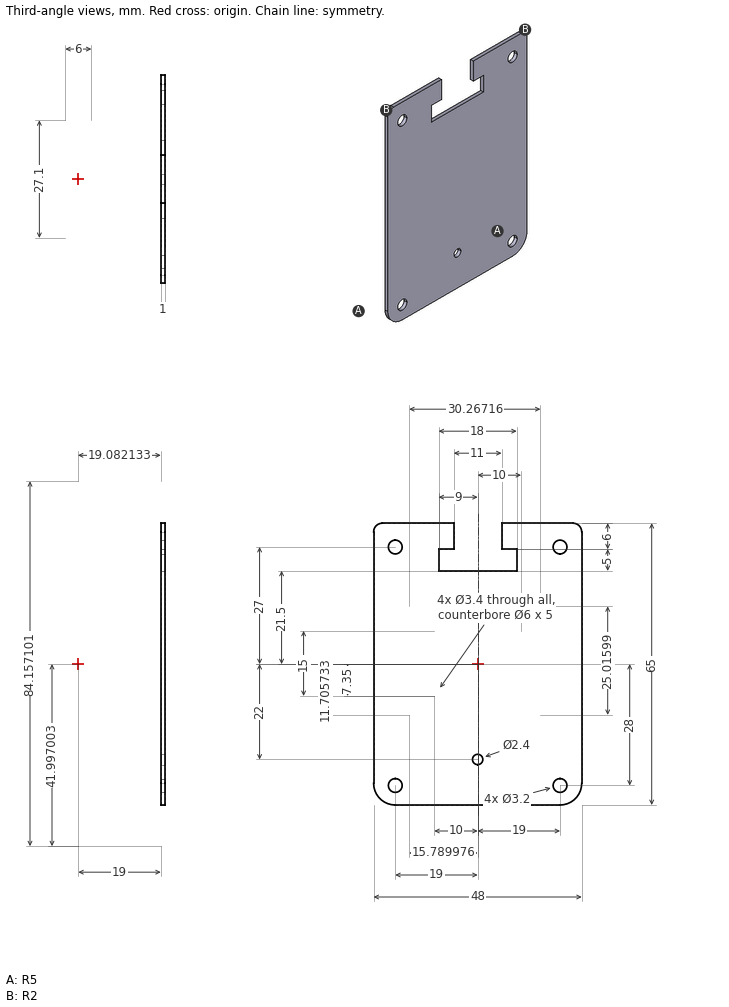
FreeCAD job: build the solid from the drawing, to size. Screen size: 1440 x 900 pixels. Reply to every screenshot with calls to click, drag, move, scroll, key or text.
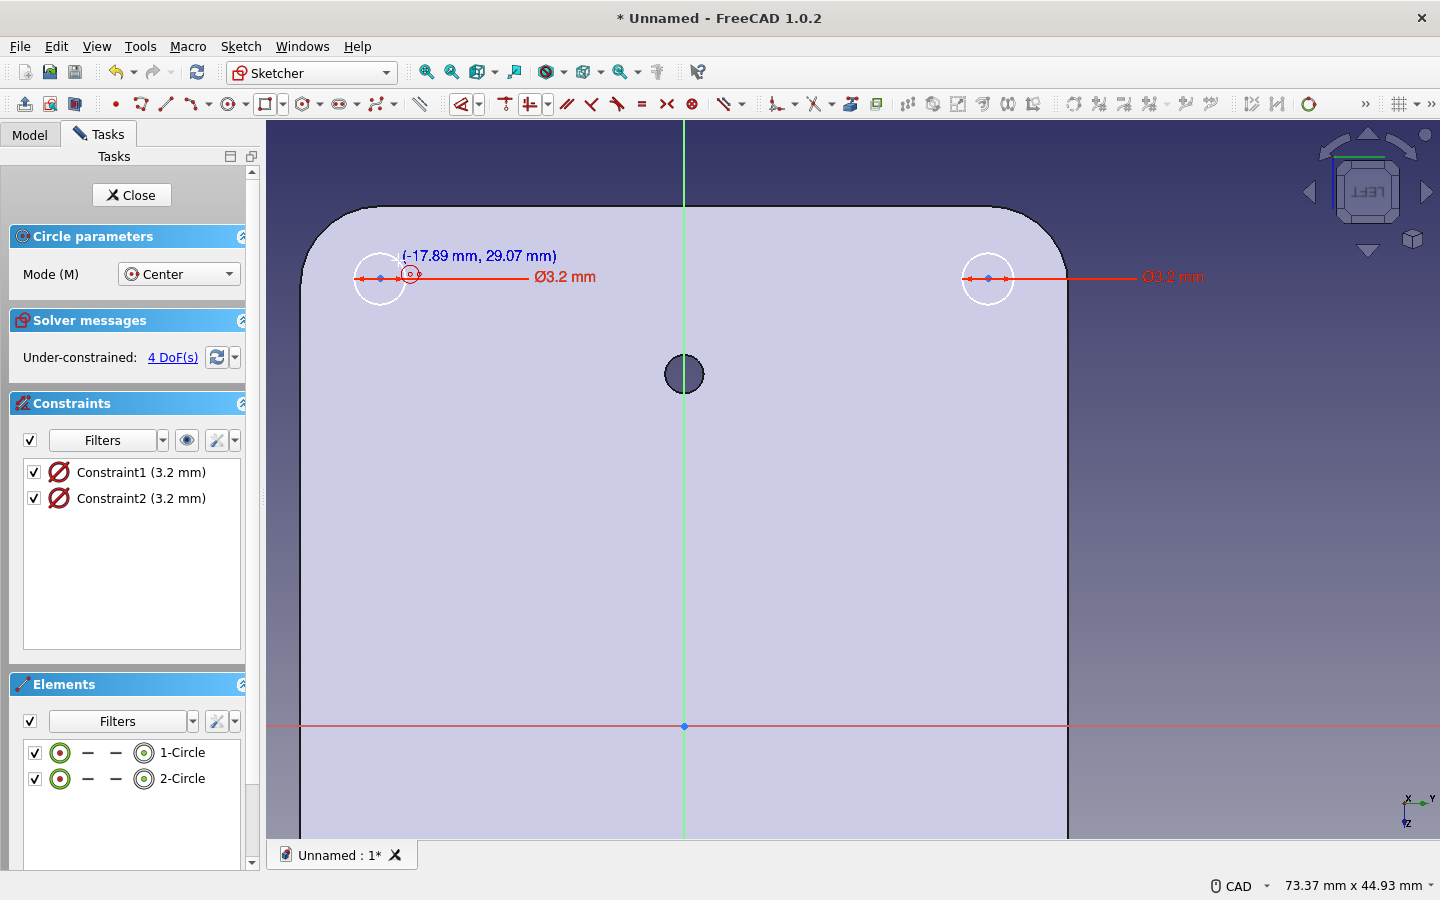
scroll(906, 189, down, 3)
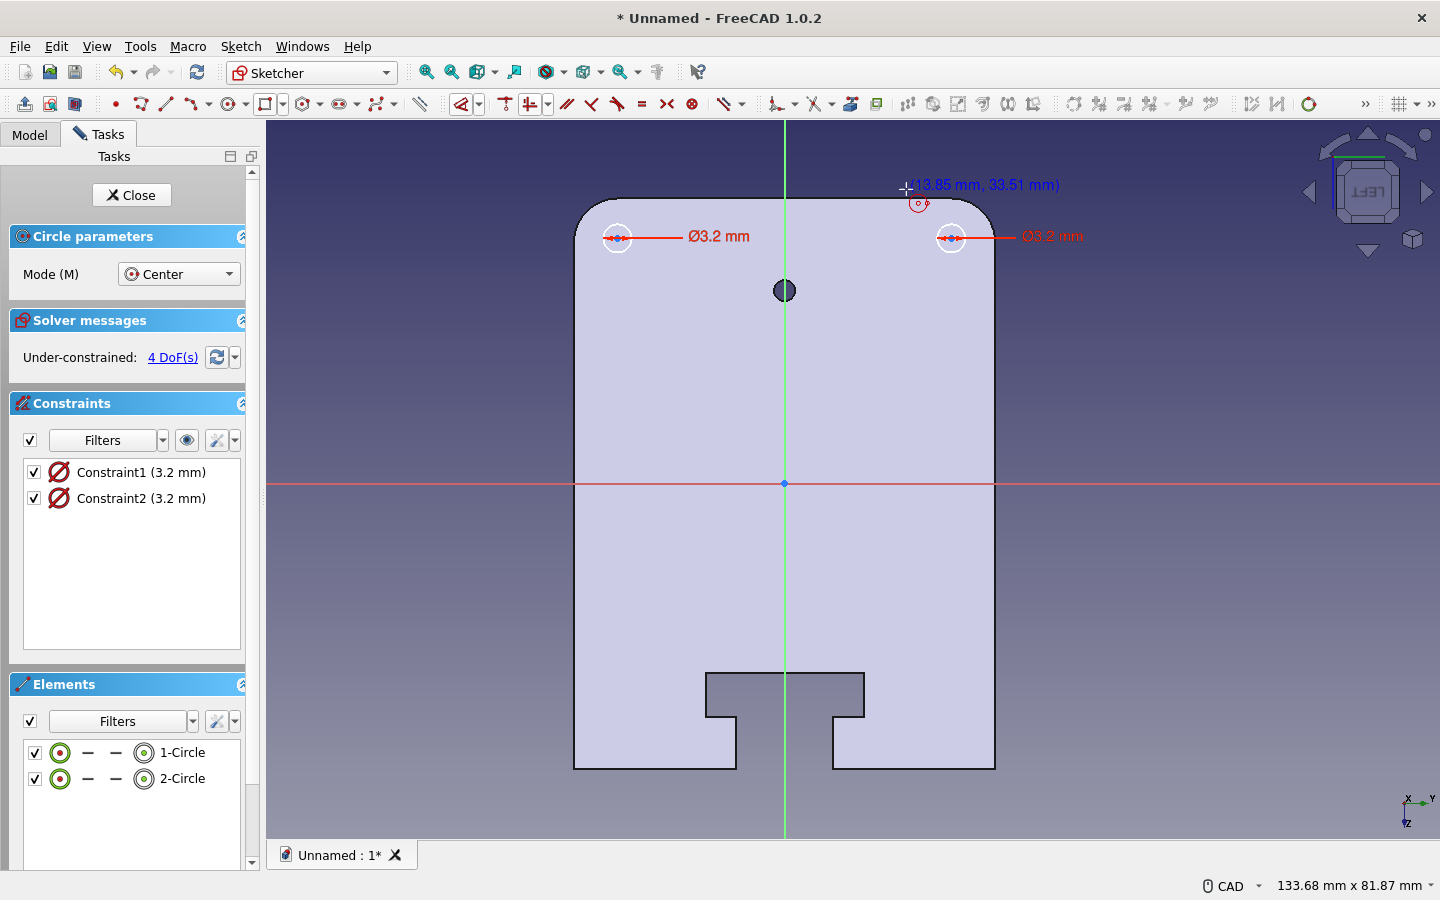
scroll(618, 721, up, 3)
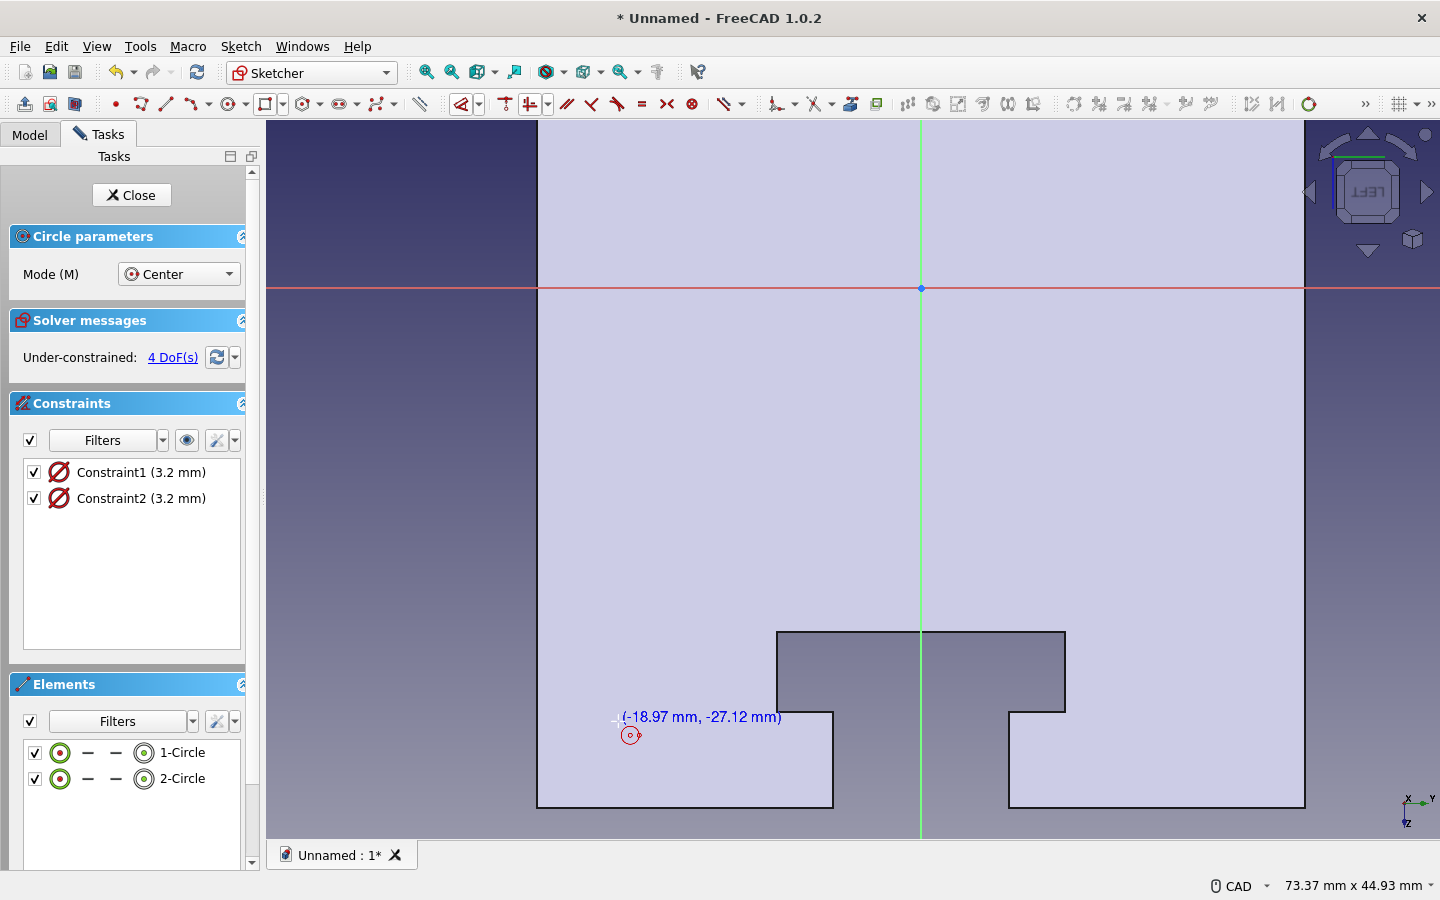
click(617, 720)
move(635, 702)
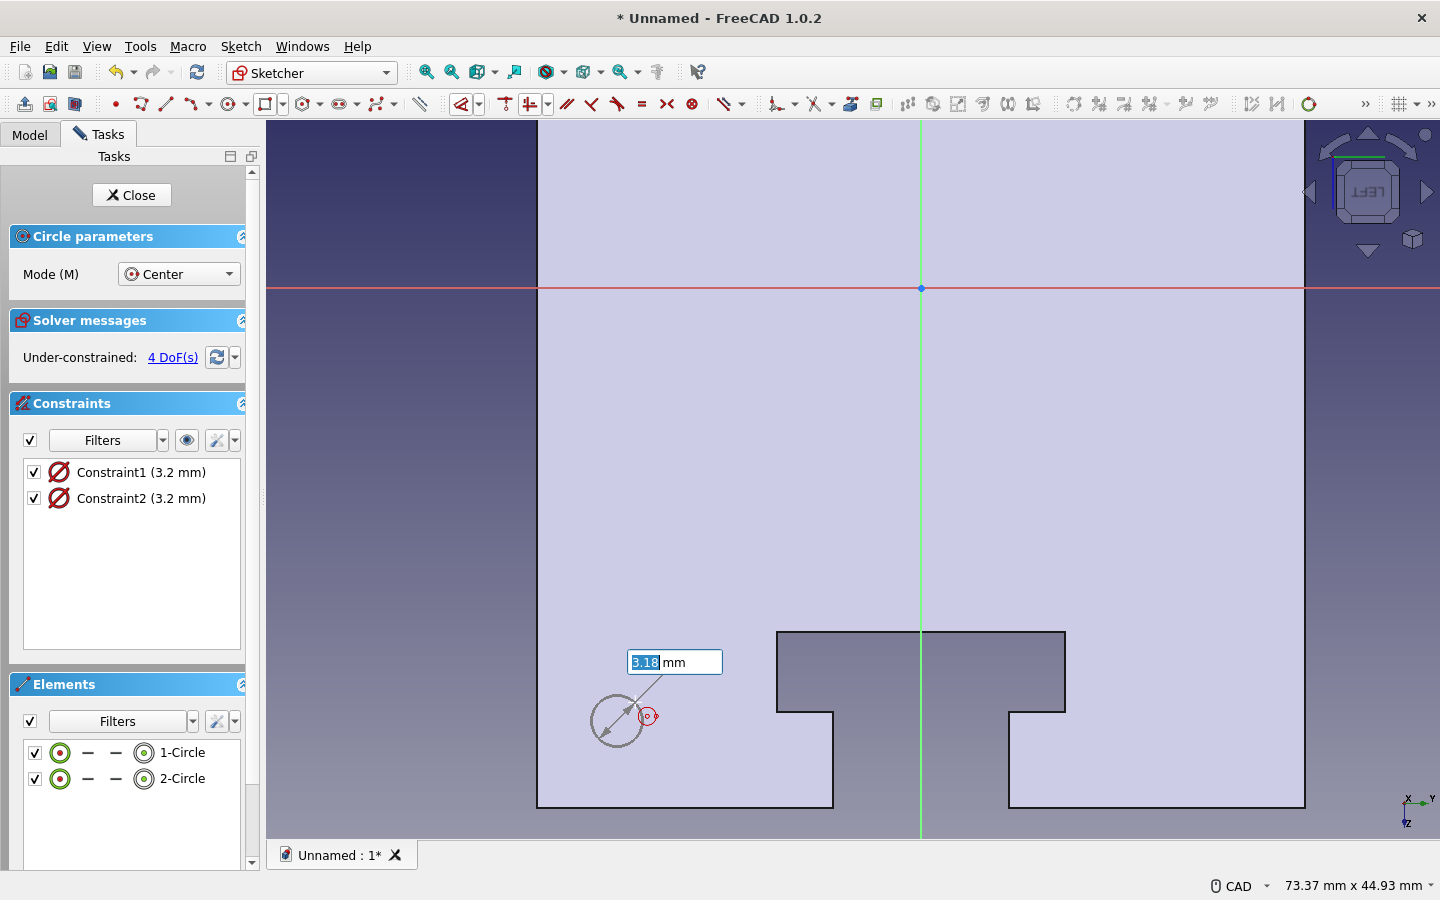
text(3.2)
key(Return)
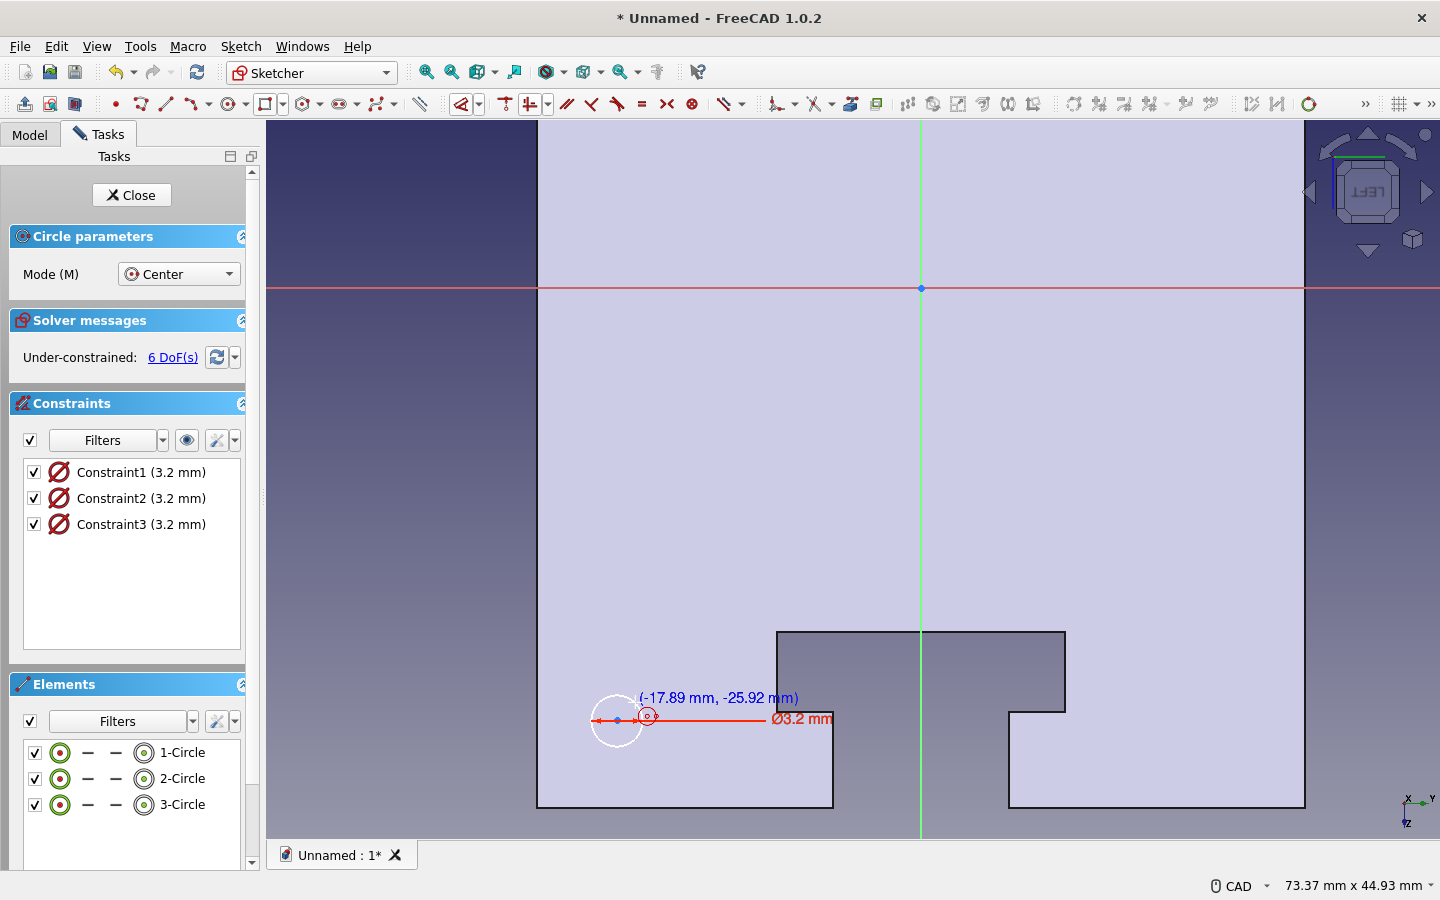
click(1225, 720)
move(1243, 702)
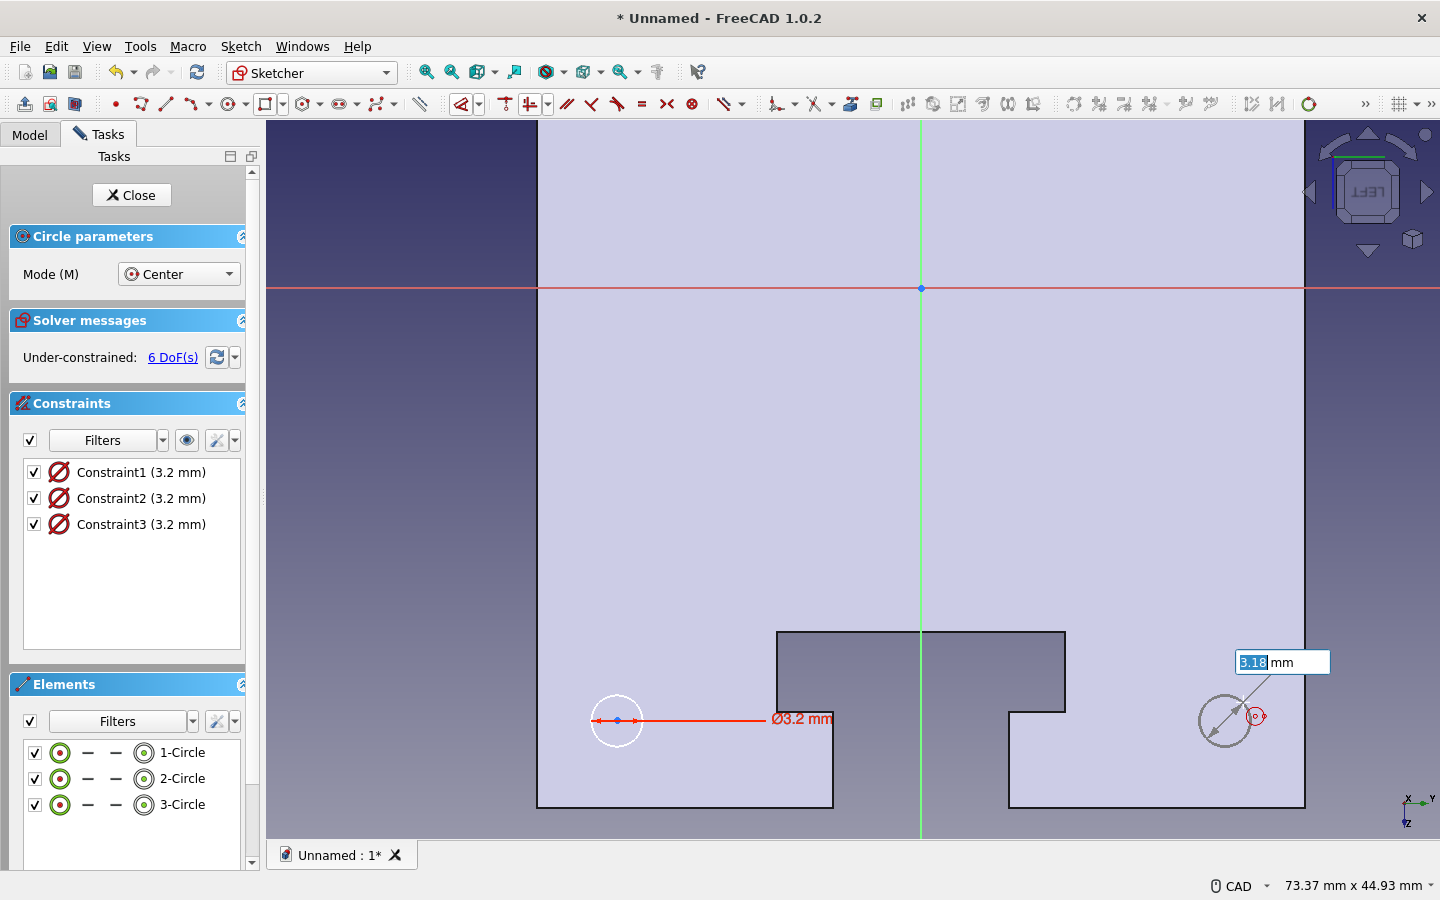
text(3.2)
key(Return)
key(Escape)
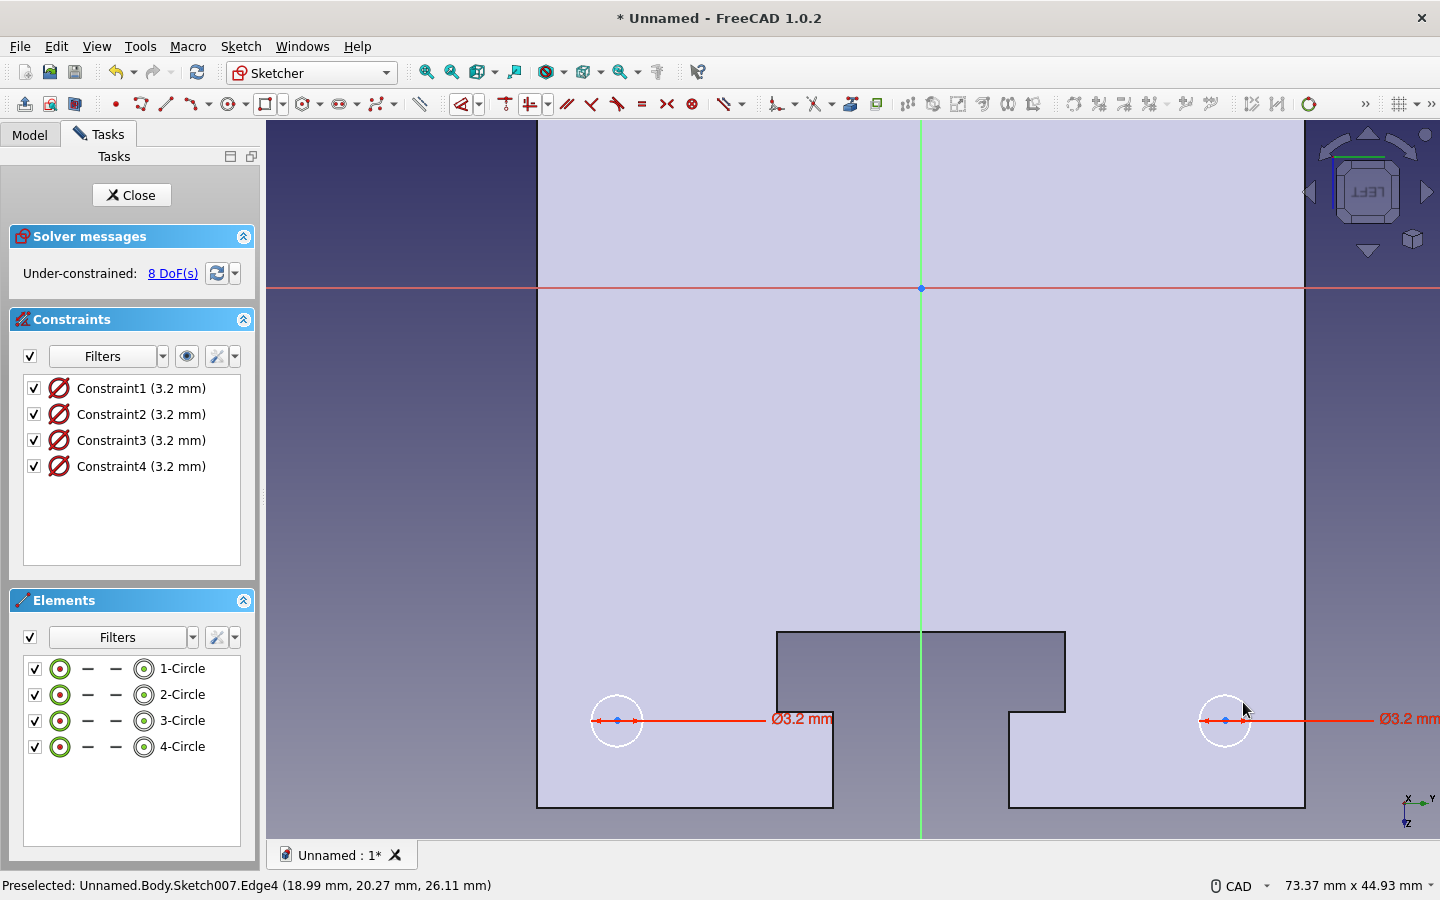
scroll(618, 722, down, 3)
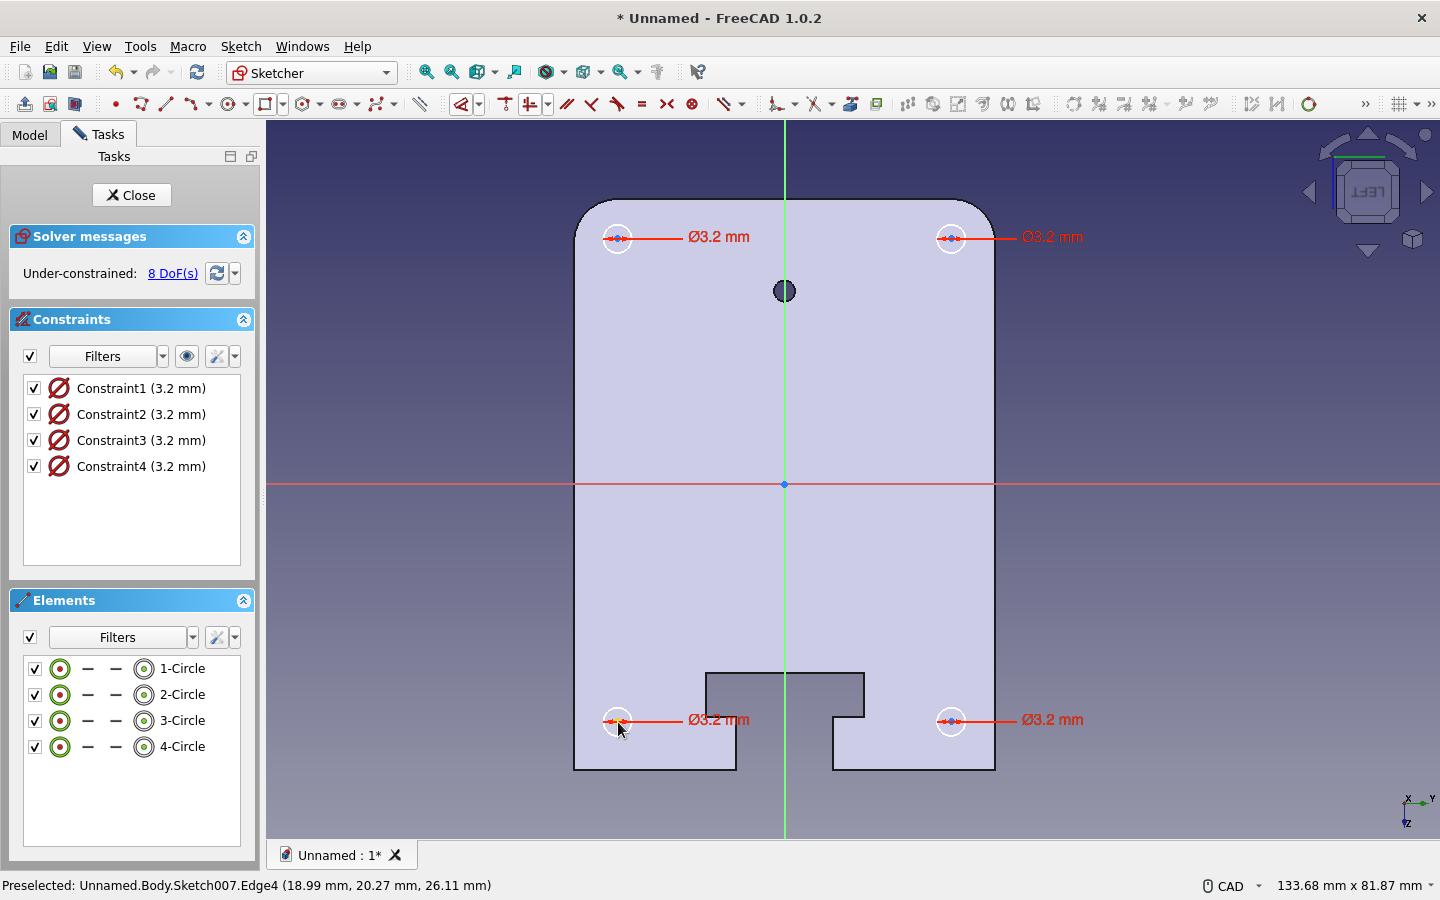
click(951, 239)